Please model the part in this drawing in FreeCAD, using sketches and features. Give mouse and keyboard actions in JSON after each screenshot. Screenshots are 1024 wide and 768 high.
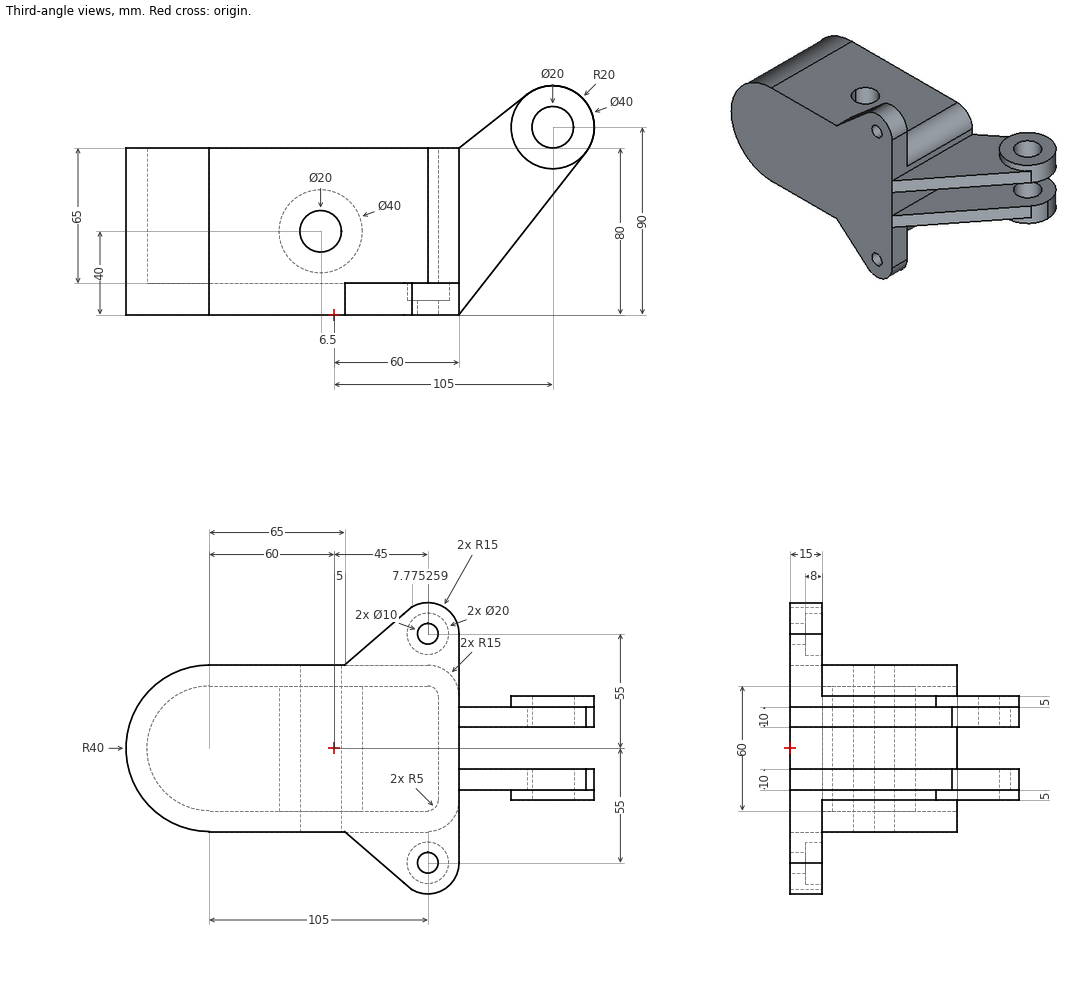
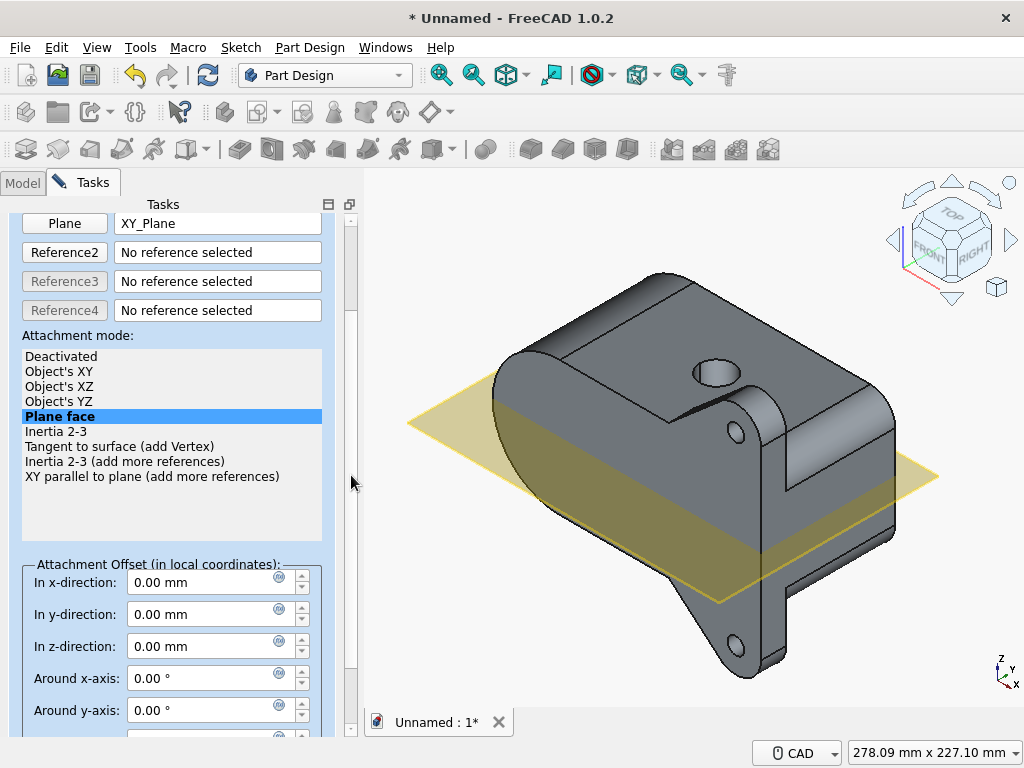
{"action": "triple_click", "coordinate": [210, 646]}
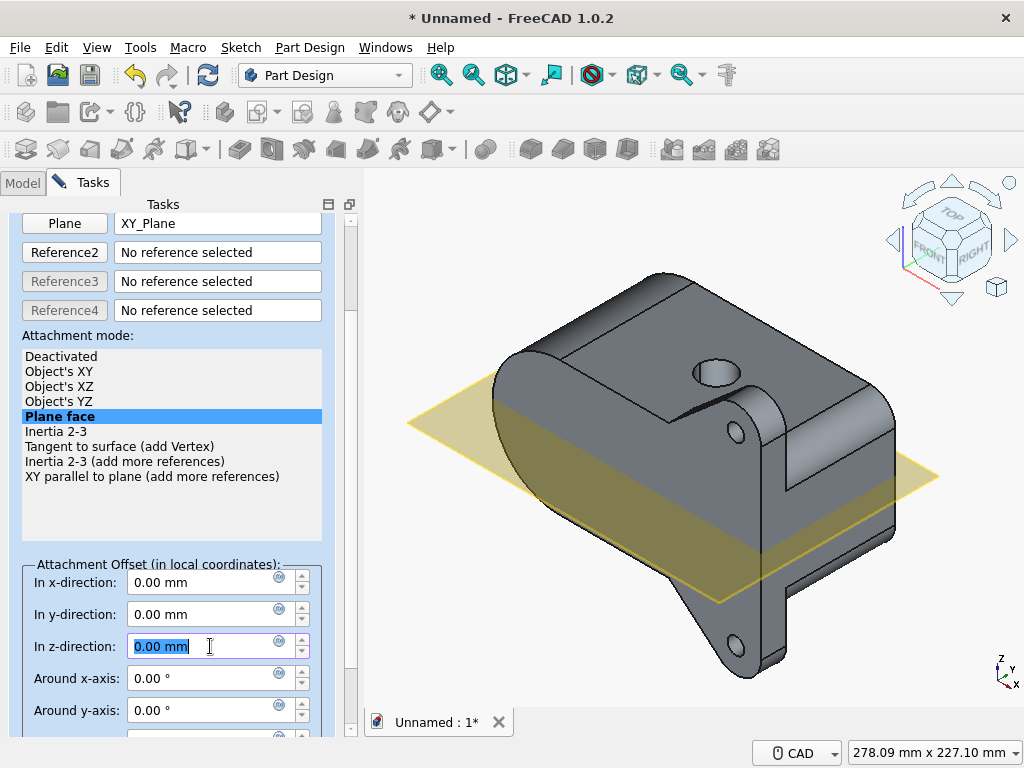
{"action": "type", "text": "10"}
{"action": "key", "text": "Tab"}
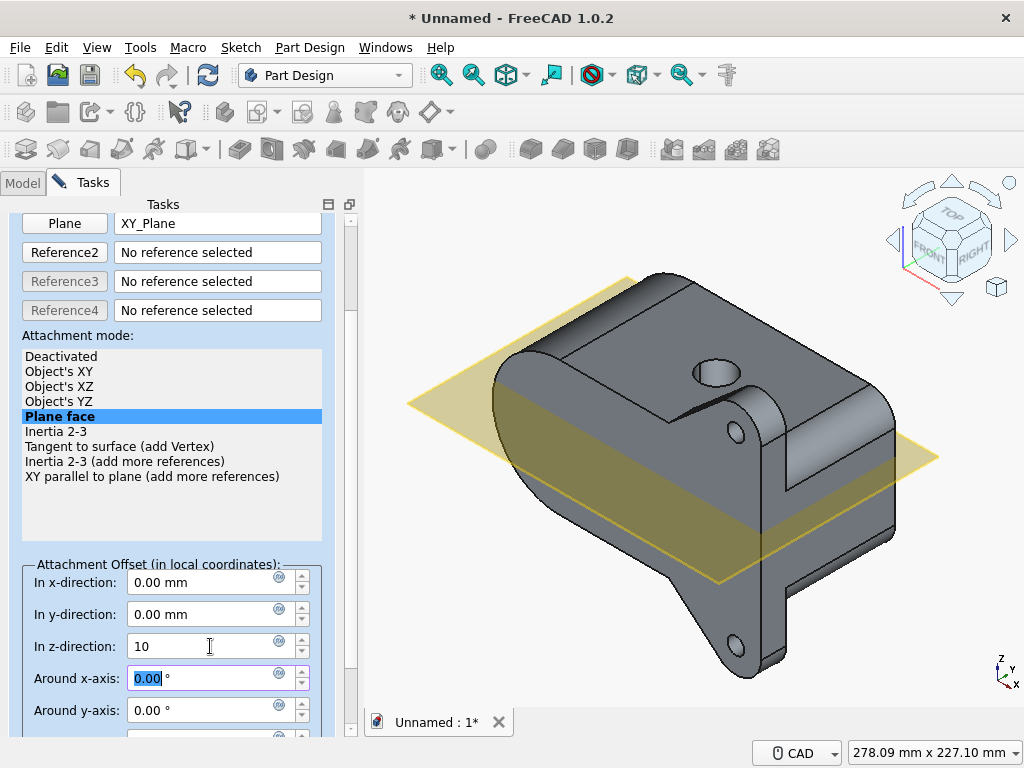
{"action": "scroll", "coordinate": [351, 475], "scroll_direction": "up", "scroll_amount": 3}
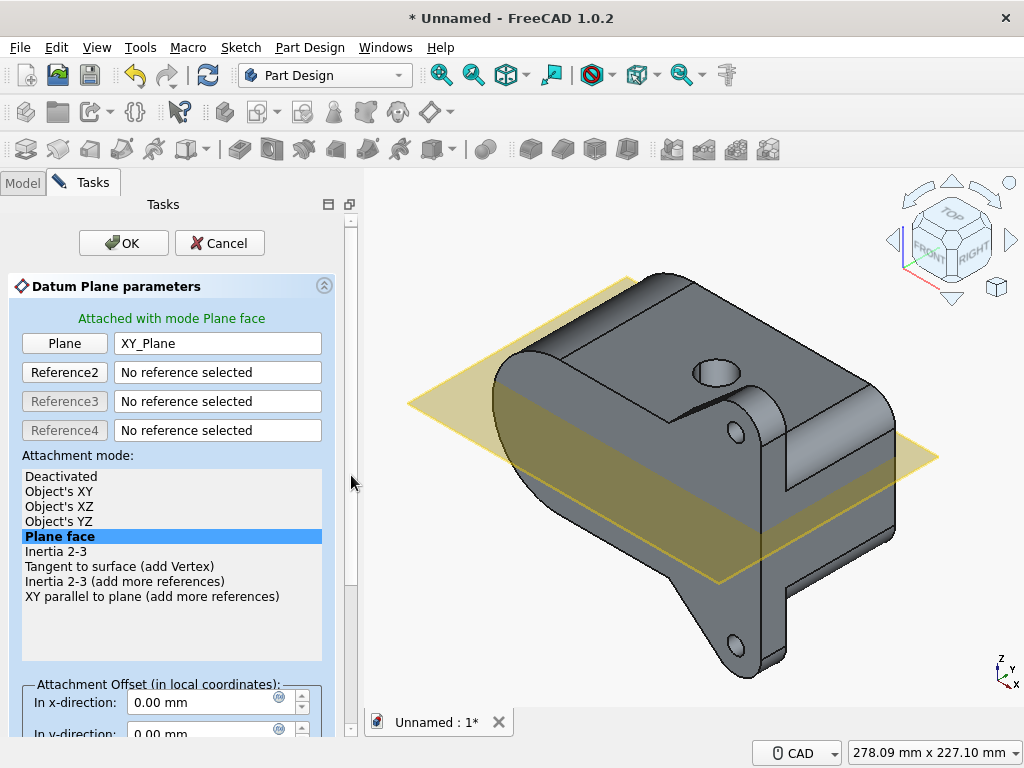
{"action": "left_click", "coordinate": [124, 243]}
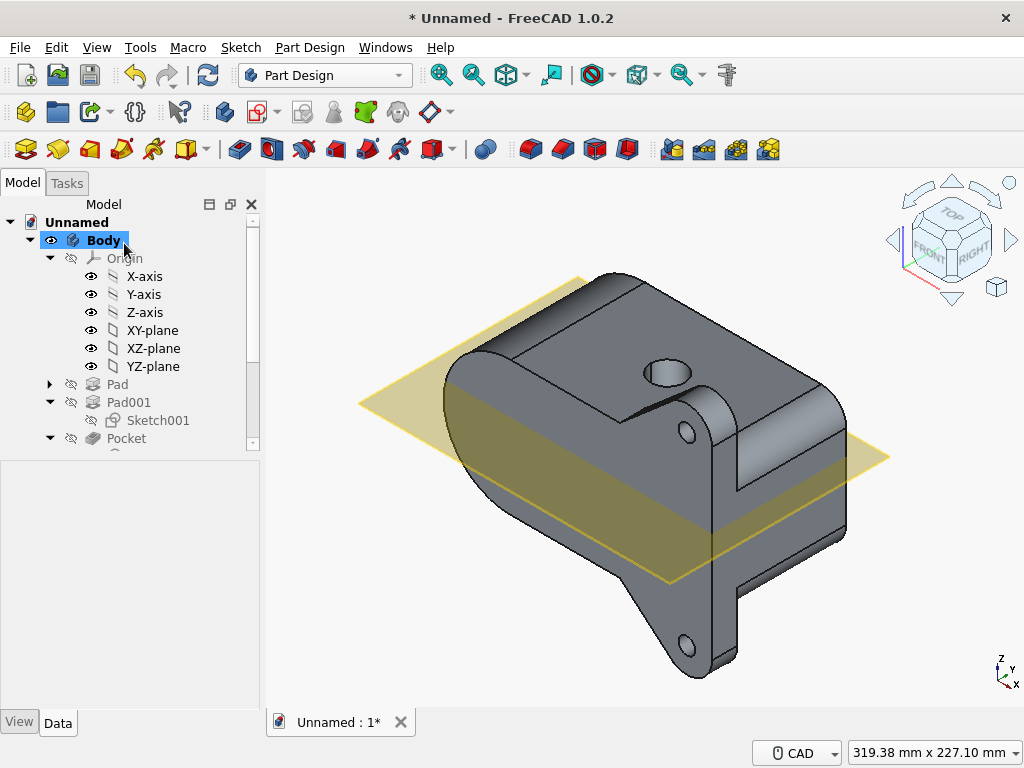
{"action": "scroll", "coordinate": [100, 326], "scroll_direction": "down", "scroll_amount": 3}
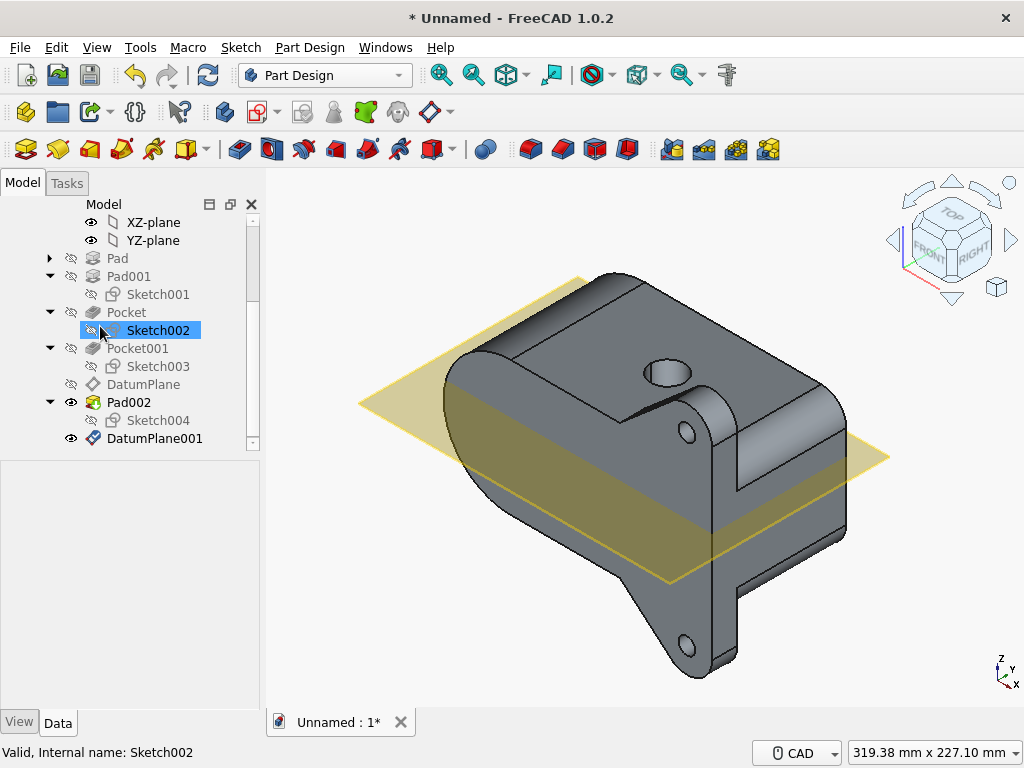
{"action": "left_click", "coordinate": [116, 438]}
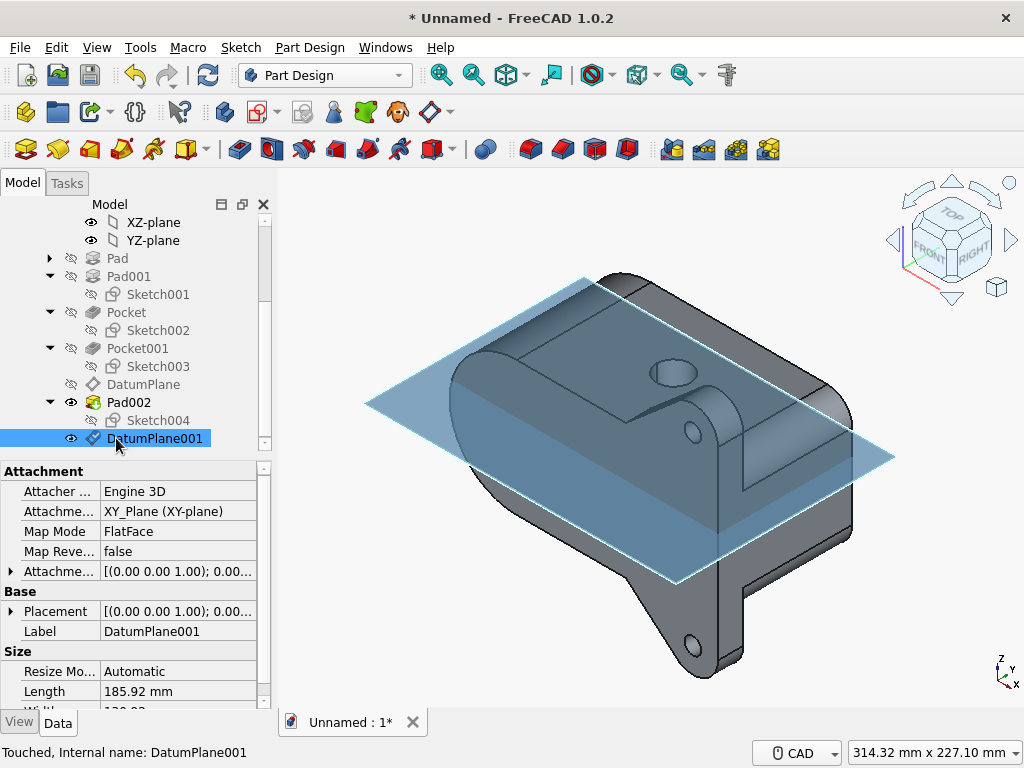
{"action": "left_click", "coordinate": [258, 112]}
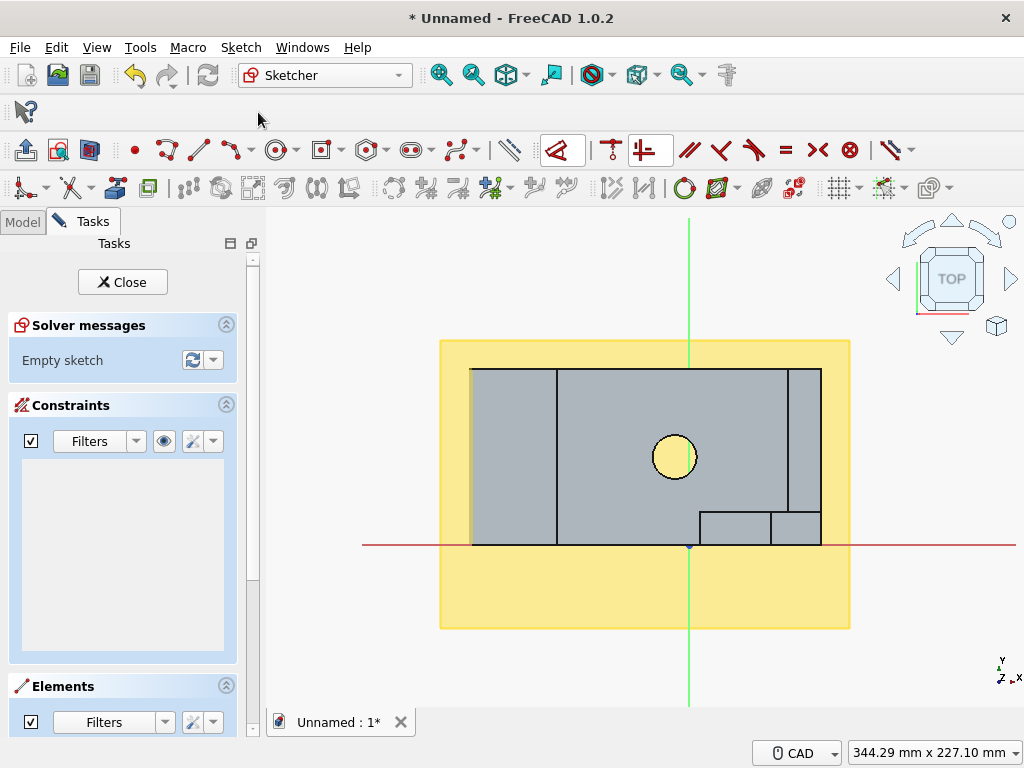
{"action": "left_click", "coordinate": [90, 150]}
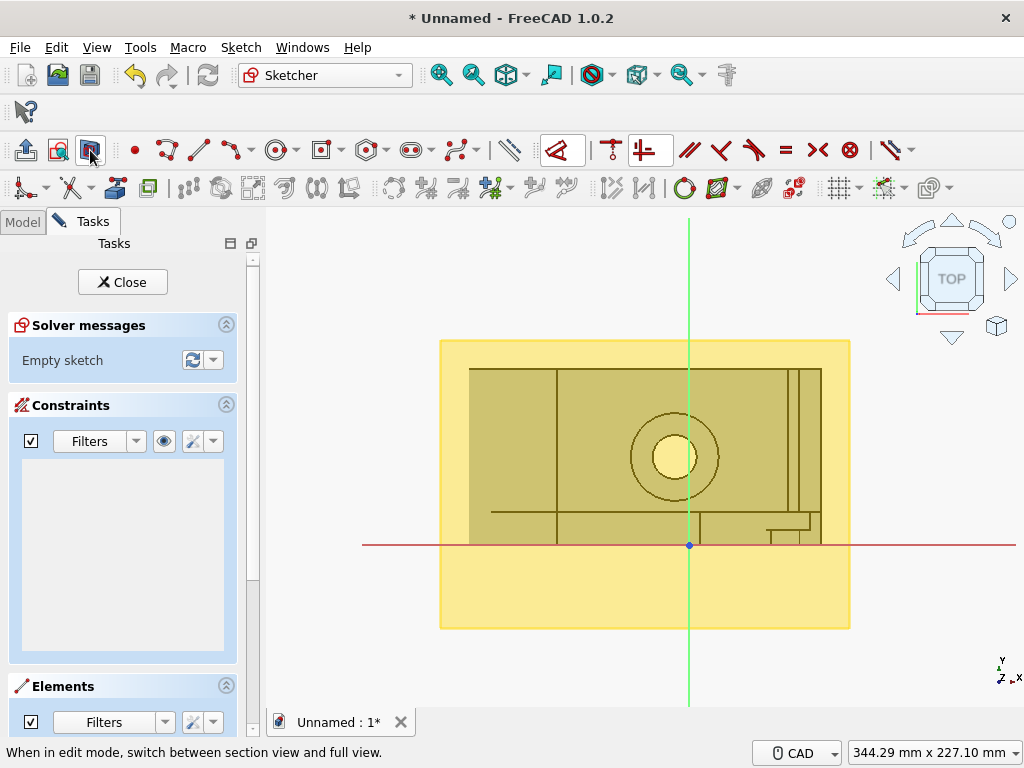
{"action": "scroll", "coordinate": [294, 515], "scroll_direction": "down", "scroll_amount": 2}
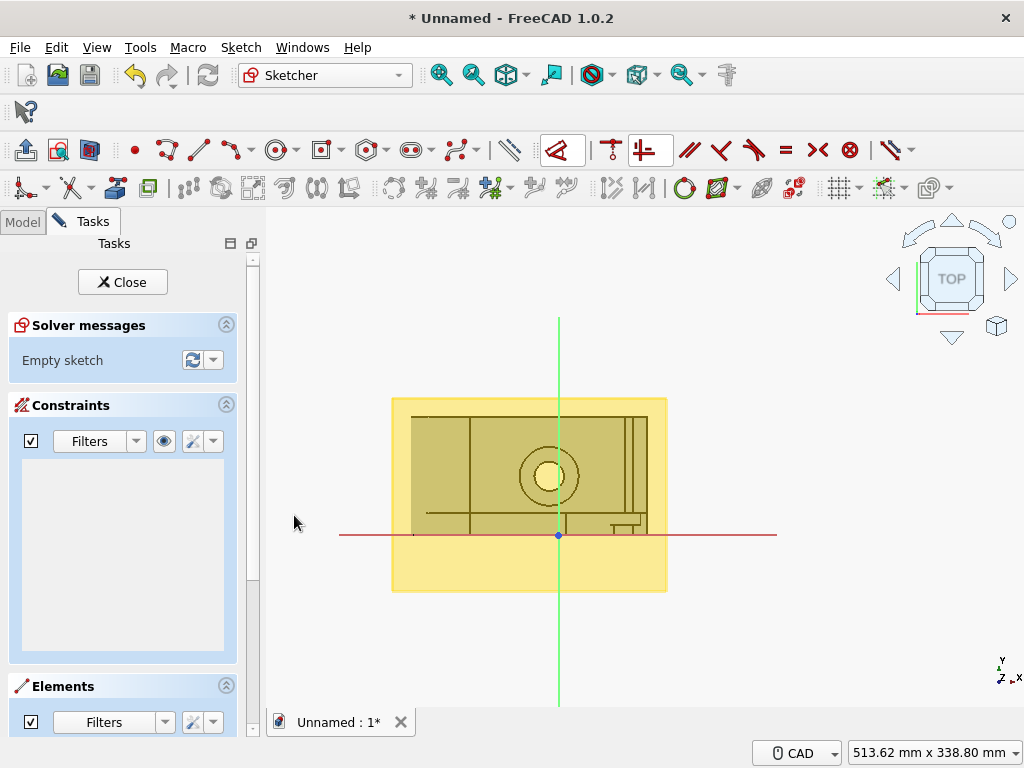
{"action": "scroll", "coordinate": [735, 458], "scroll_direction": "up", "scroll_amount": 3}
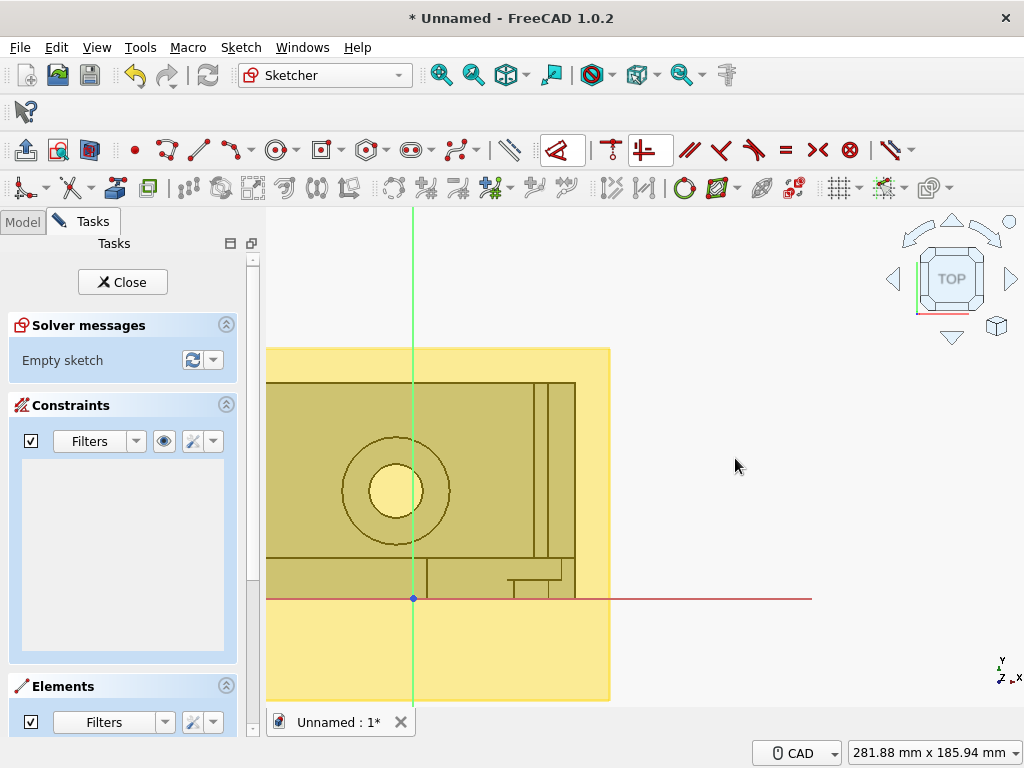
{"action": "left_click", "coordinate": [168, 150]}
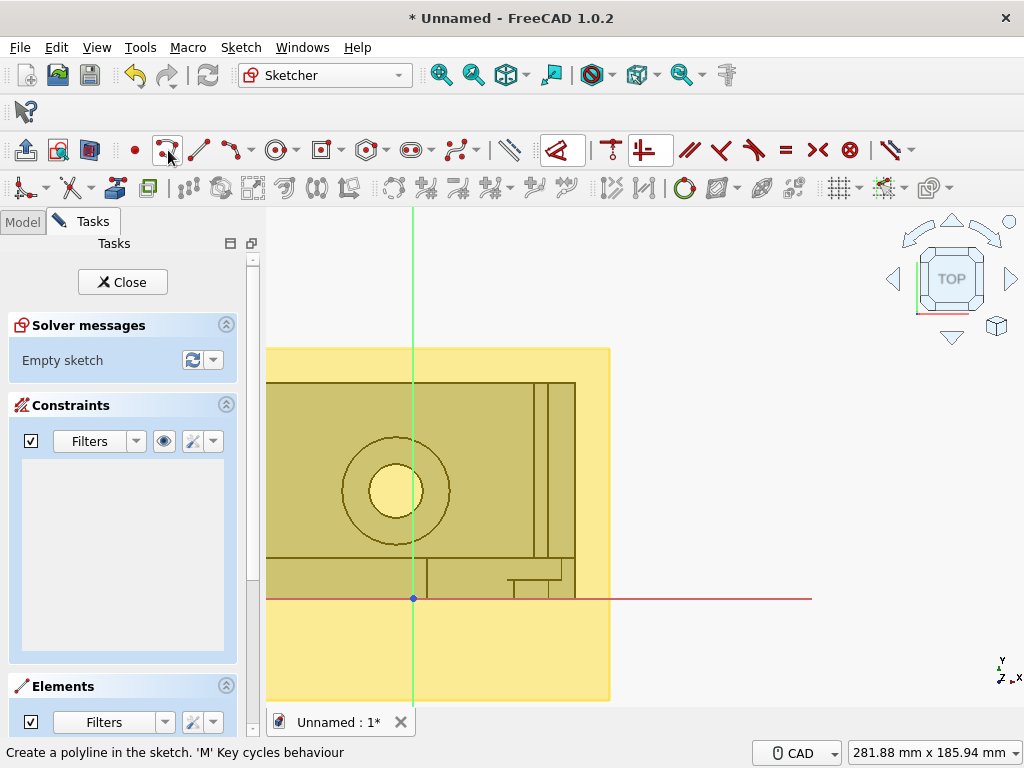
{"action": "left_click", "coordinate": [663, 314]}
{"action": "left_click", "coordinate": [575, 383]}
{"action": "left_click", "coordinate": [575, 599]}
{"action": "left_click", "coordinate": [738, 390]}
{"action": "right_click", "coordinate": [738, 390]}